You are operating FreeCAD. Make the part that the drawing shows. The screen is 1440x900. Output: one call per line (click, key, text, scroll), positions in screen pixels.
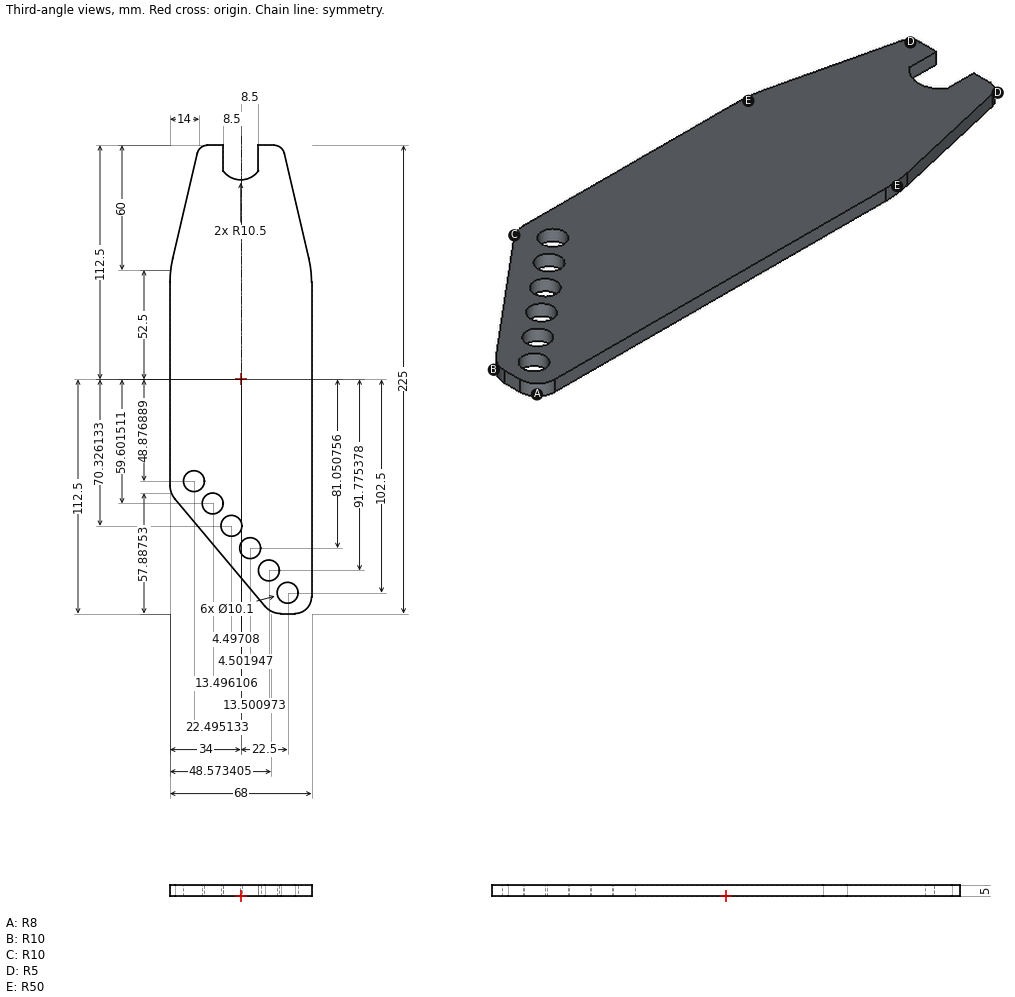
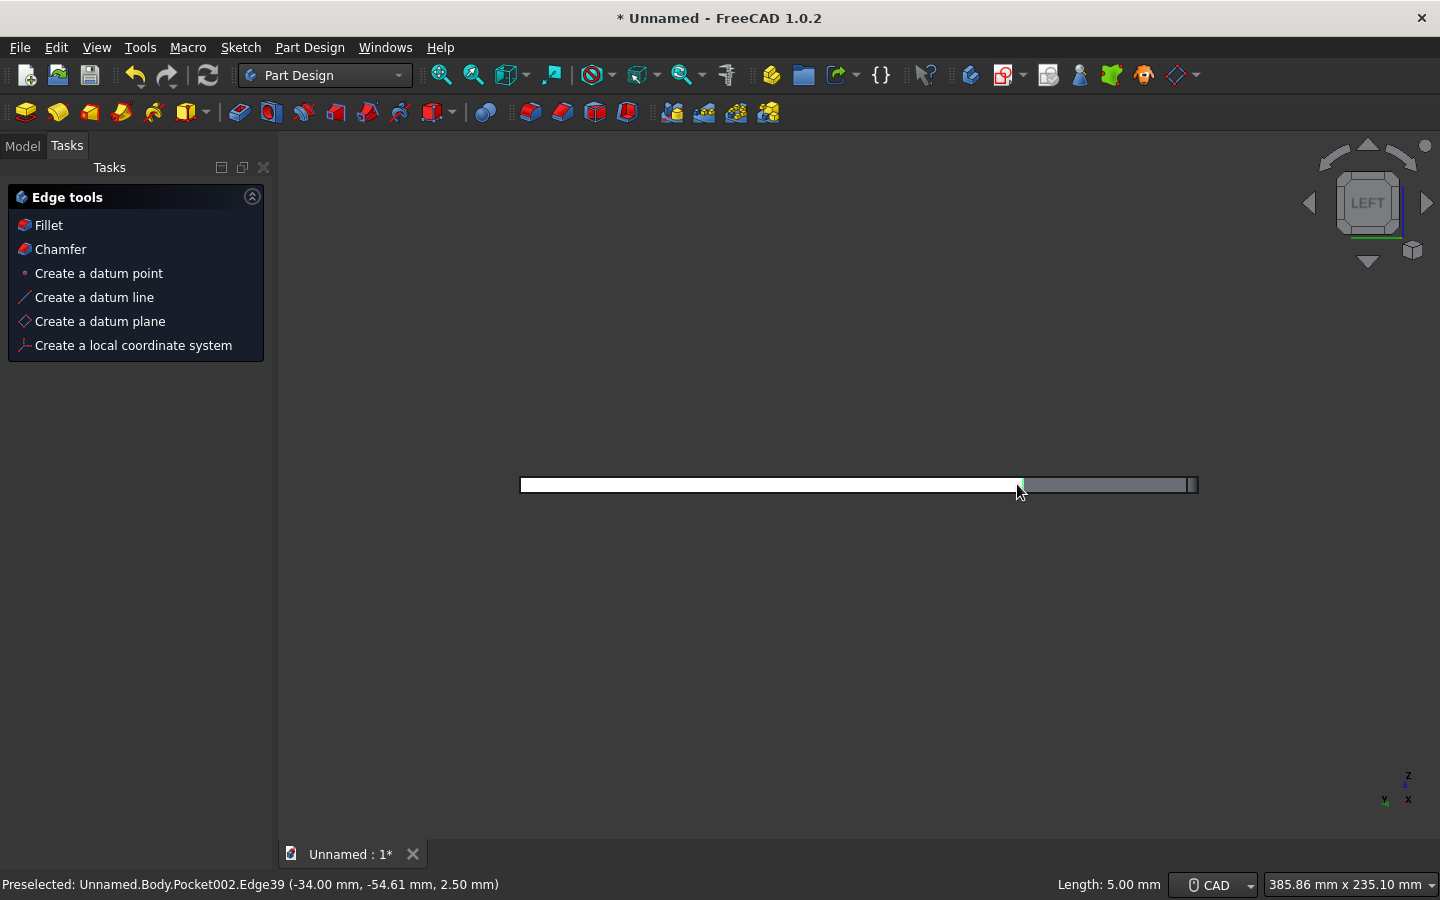
click(532, 112)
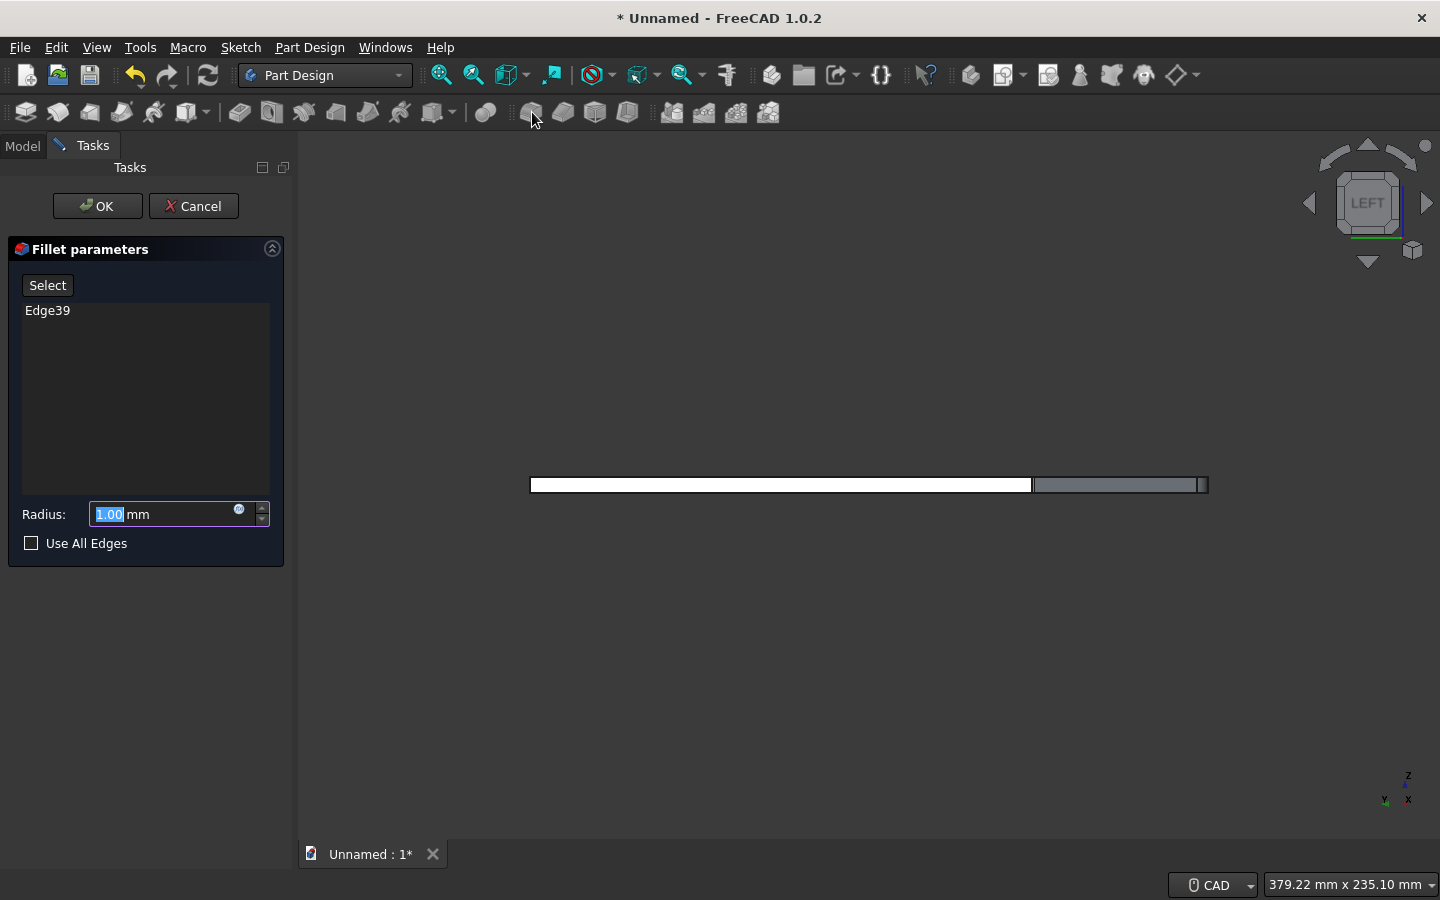
text(10)
key(Tab)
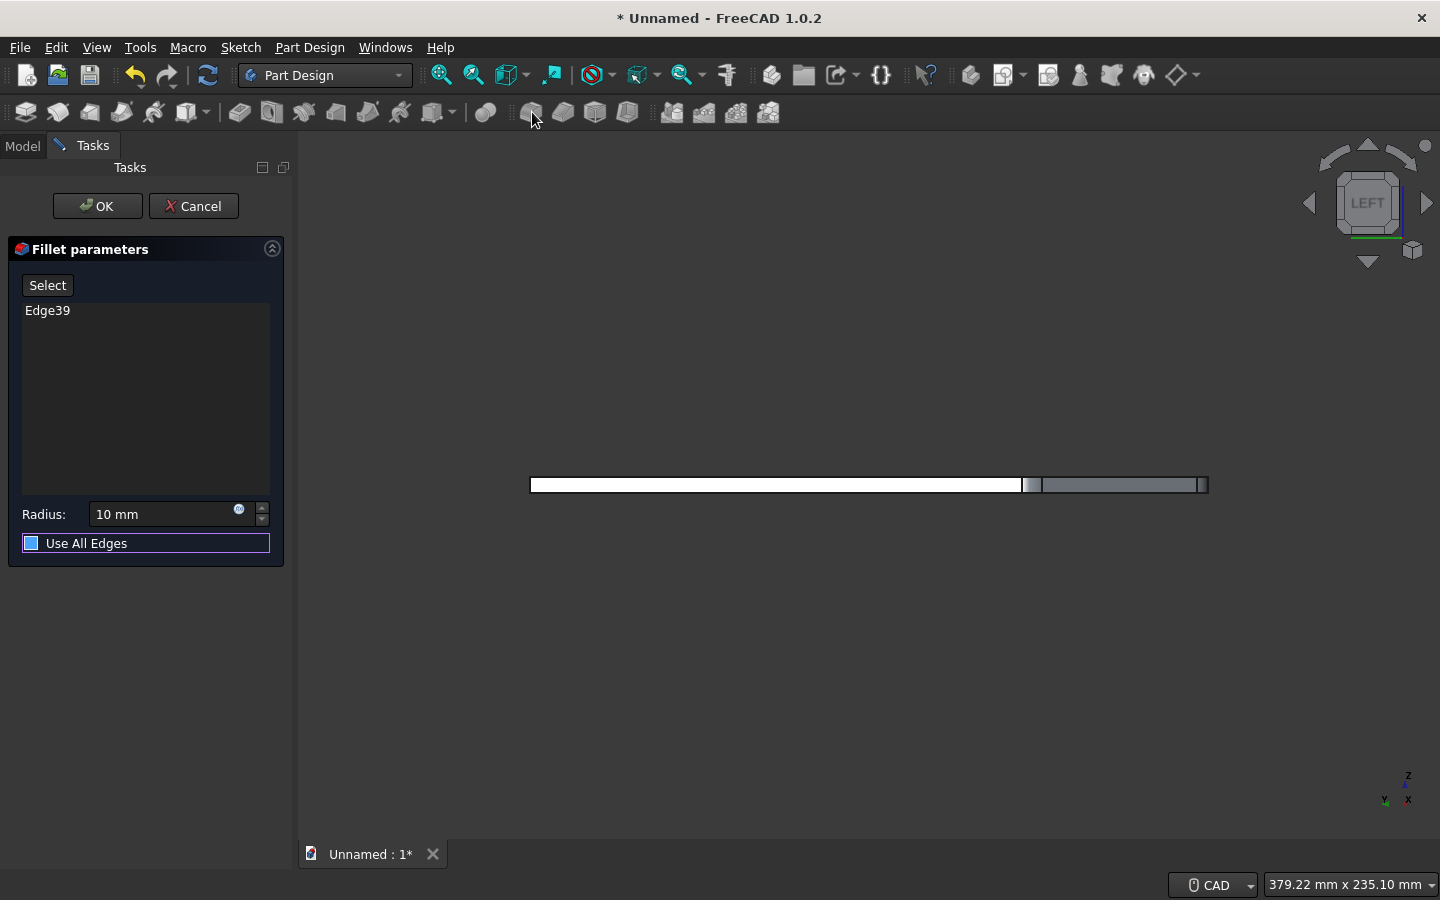
click(98, 206)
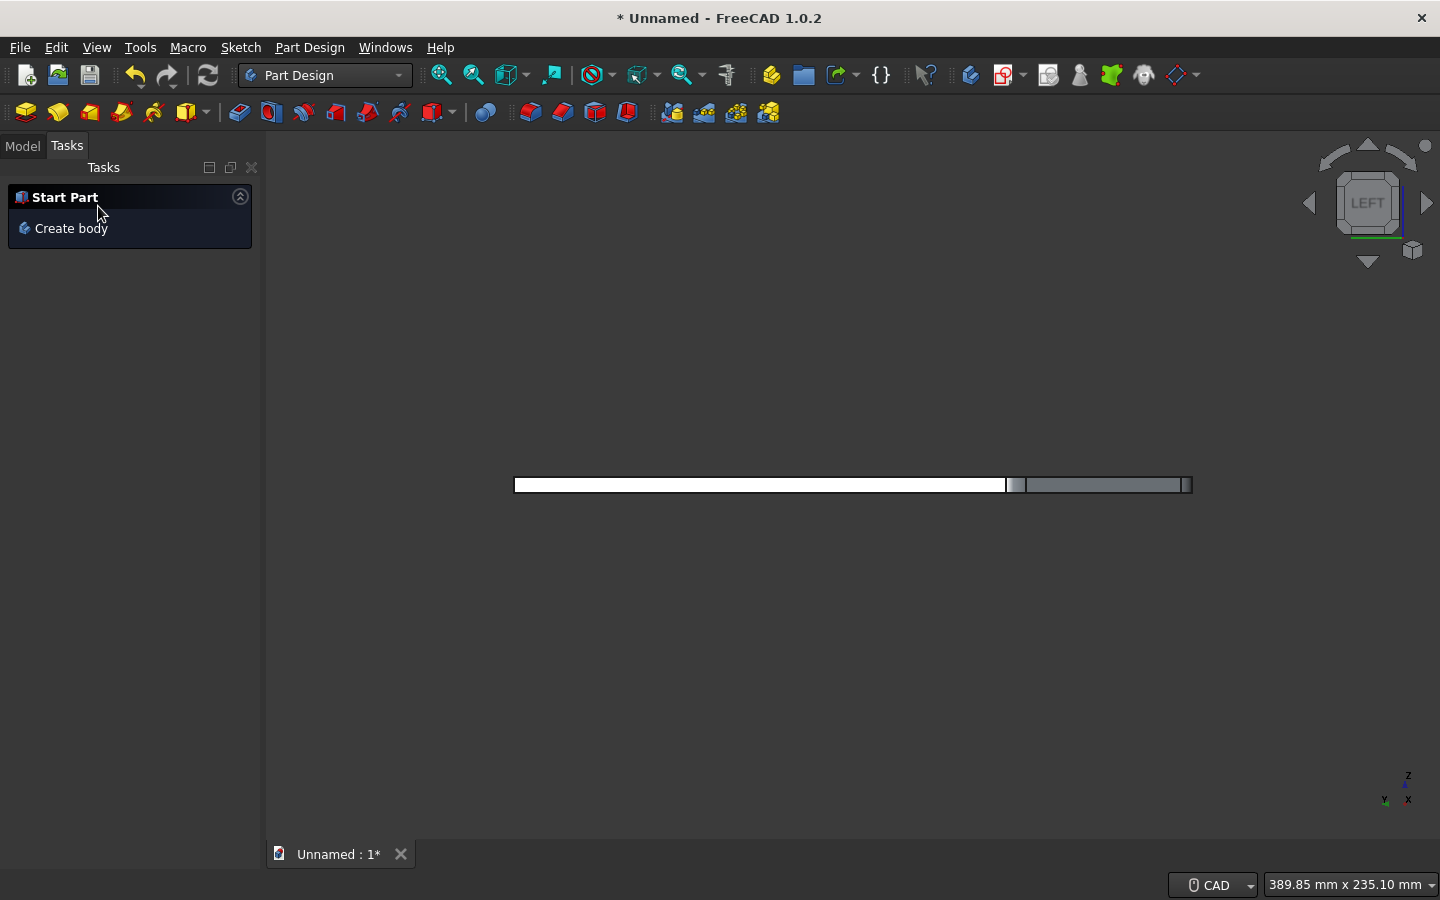
key(0)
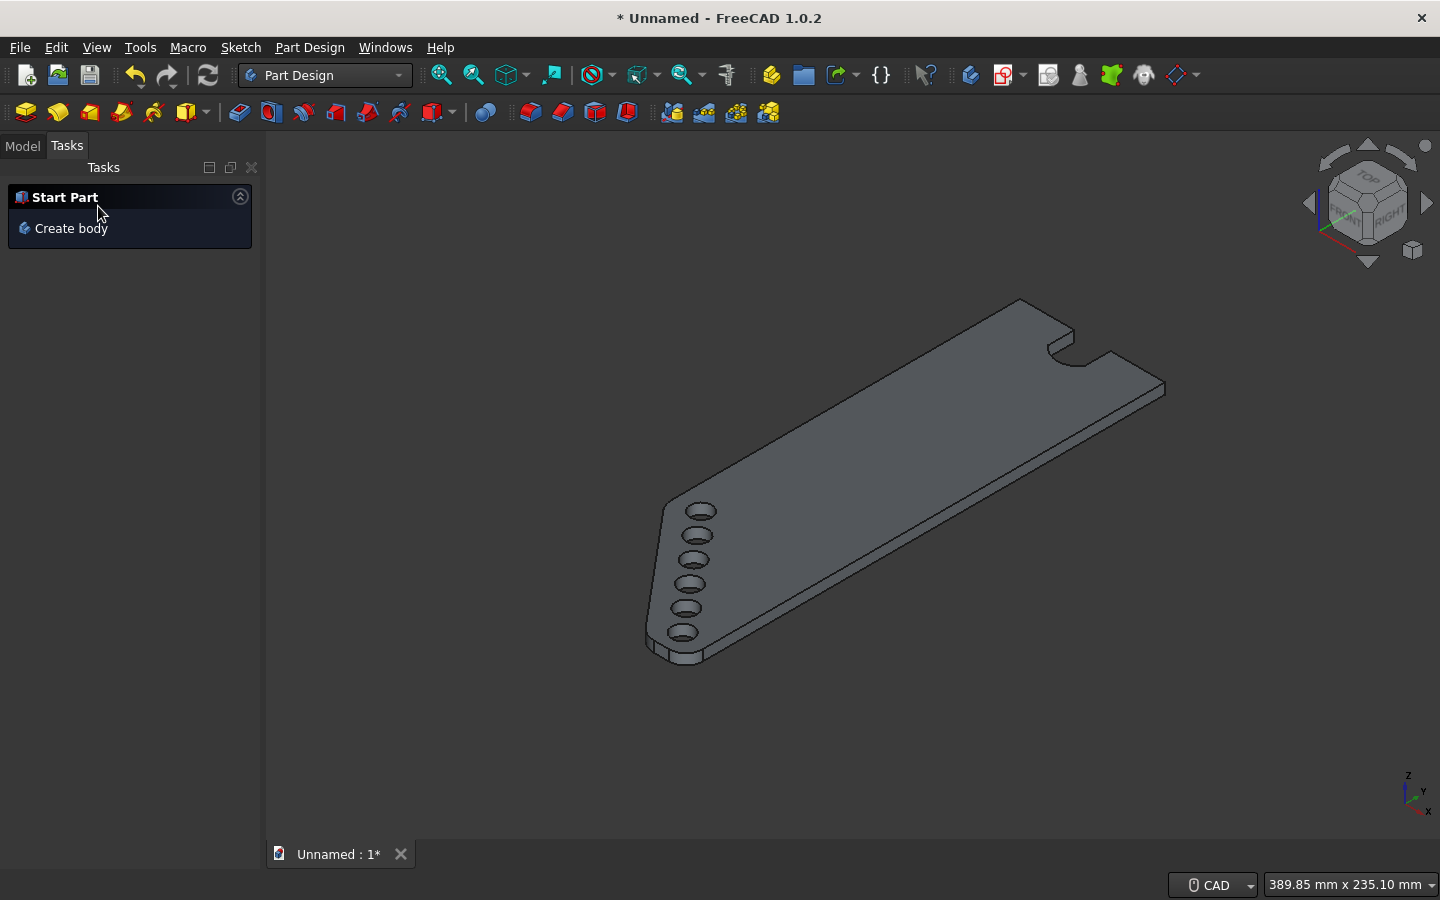
click(921, 438)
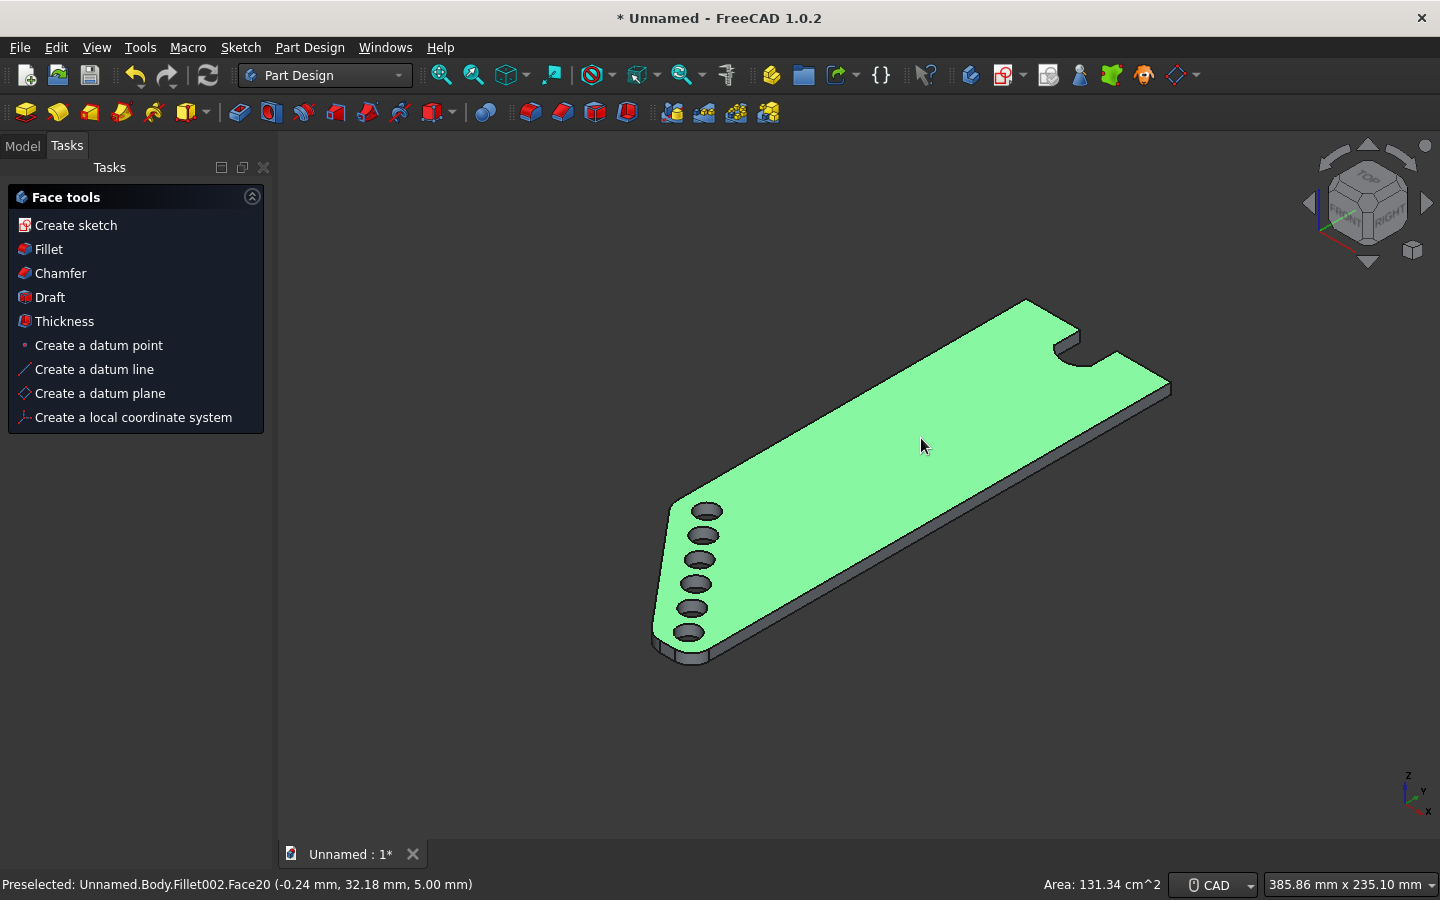
click(1004, 76)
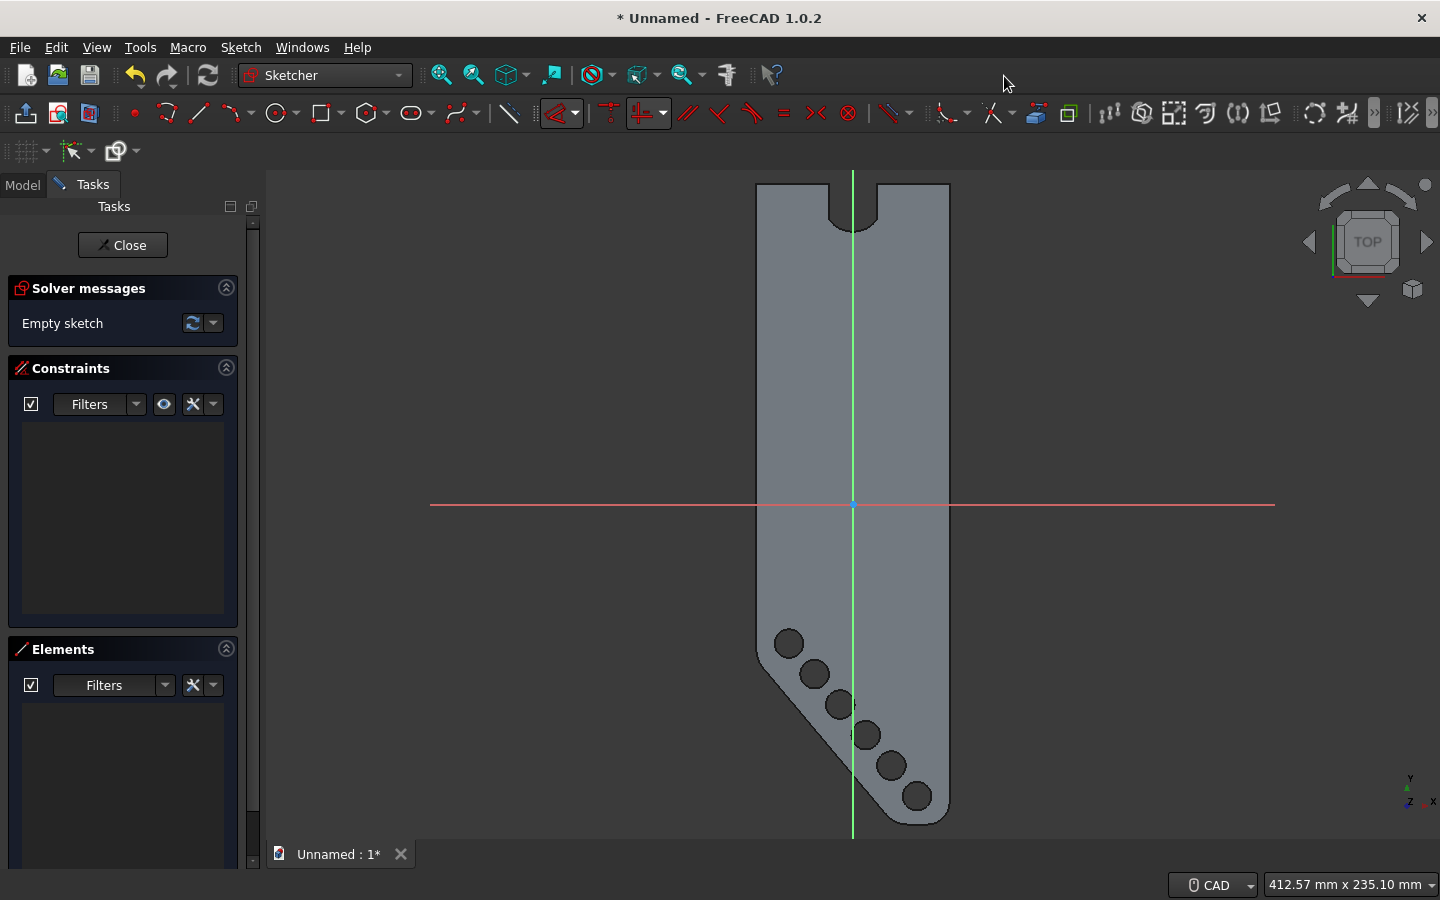
scroll(475, 811, down, 1)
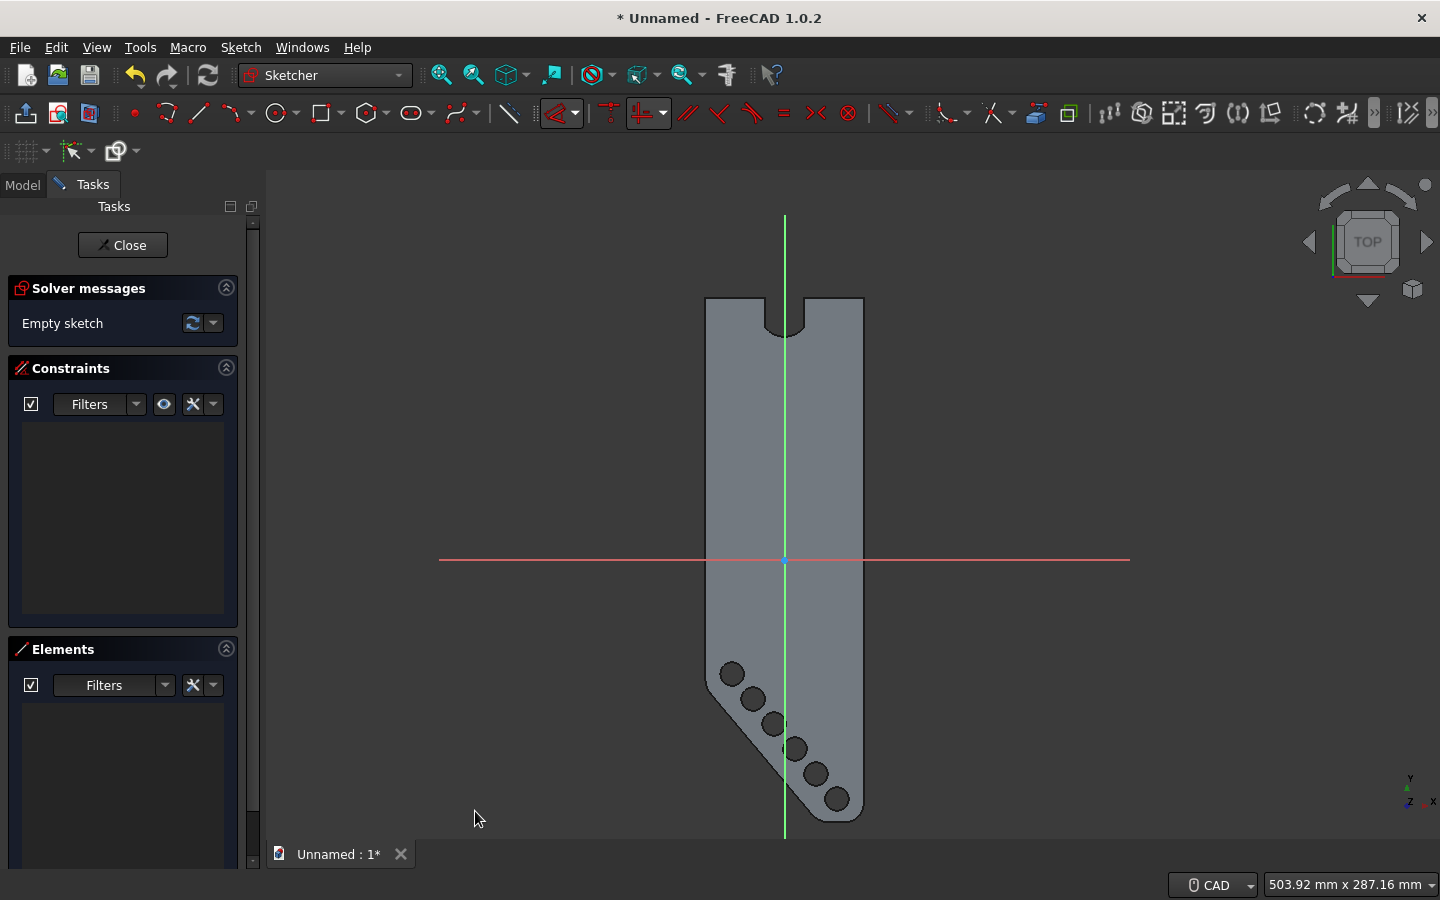
scroll(785, 338, up, 3)